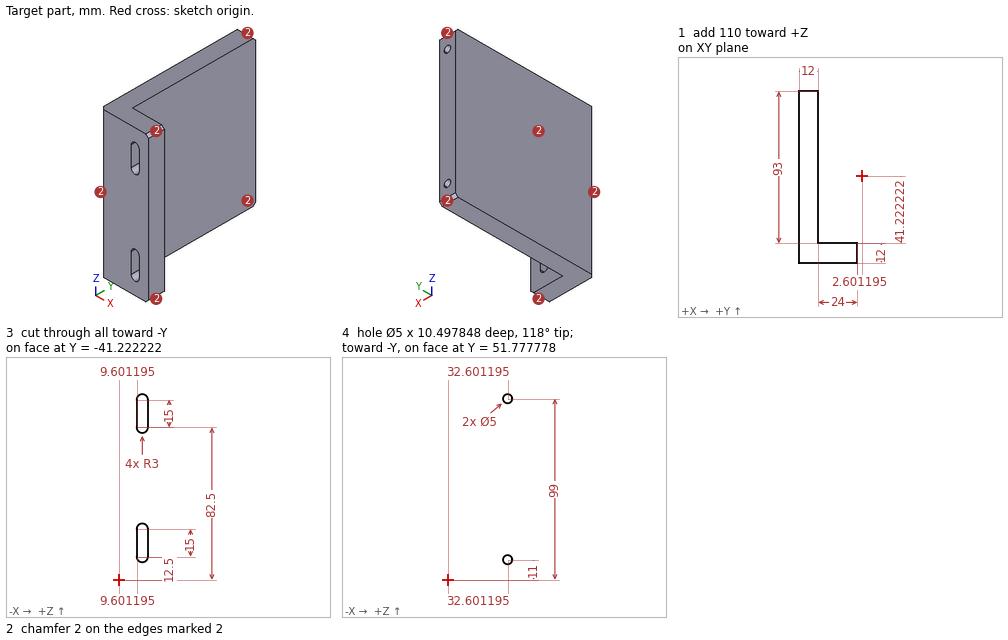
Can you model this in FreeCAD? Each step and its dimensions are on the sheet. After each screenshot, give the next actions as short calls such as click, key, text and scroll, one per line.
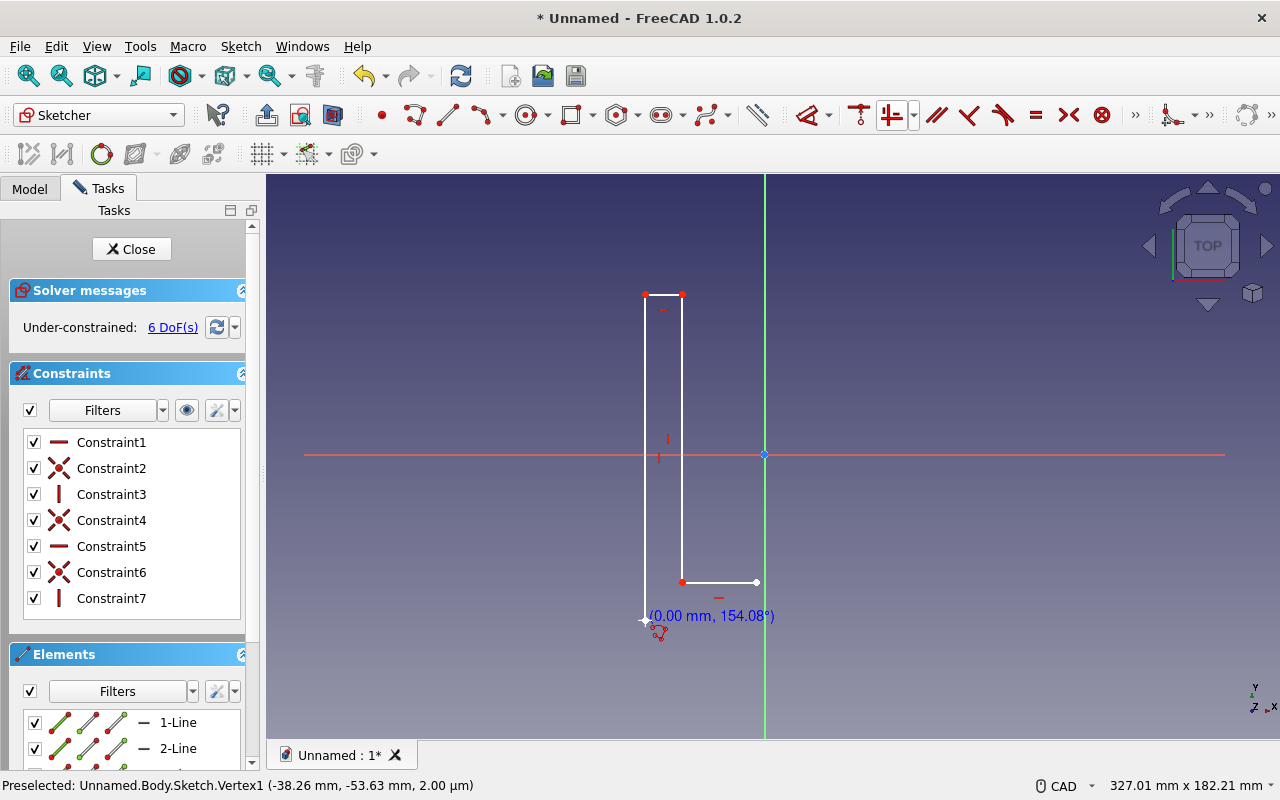
scroll(757, 620, up, 4)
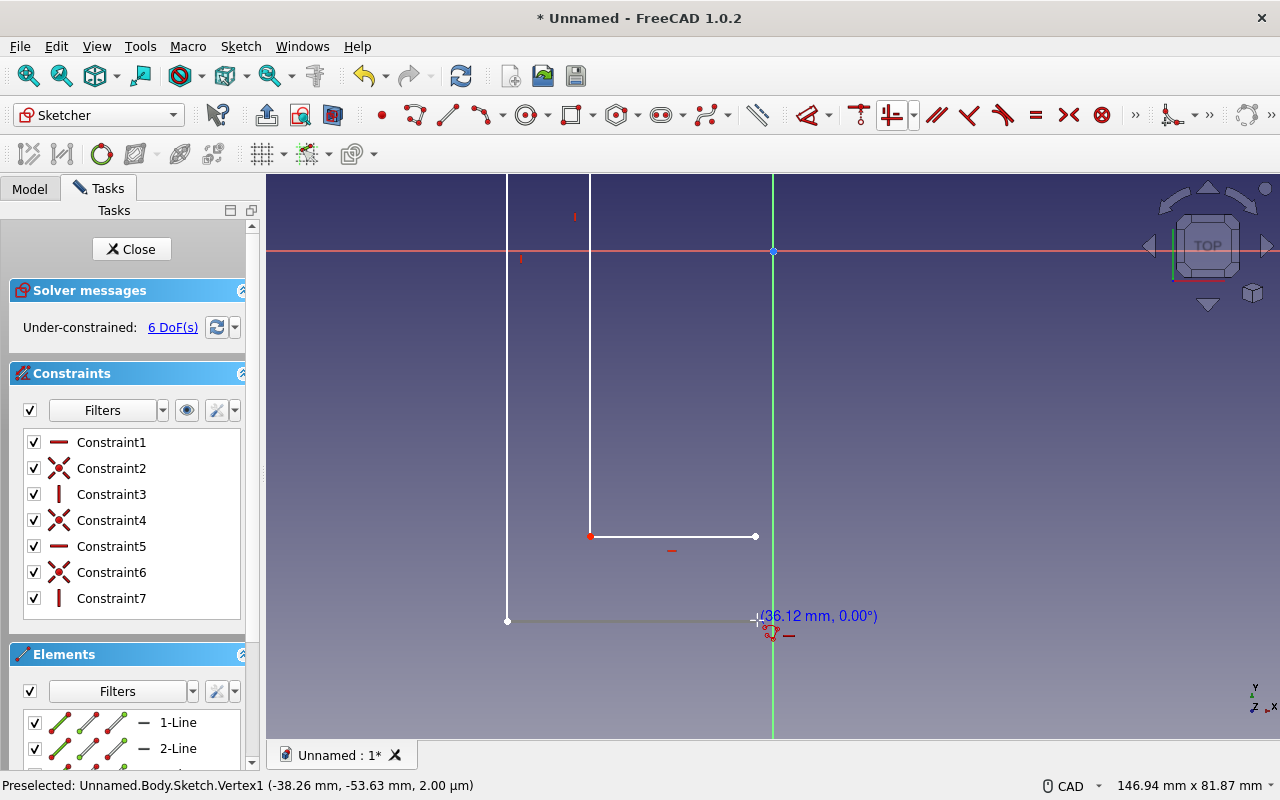
click(755, 619)
click(755, 537)
key(Escape)
key(Escape)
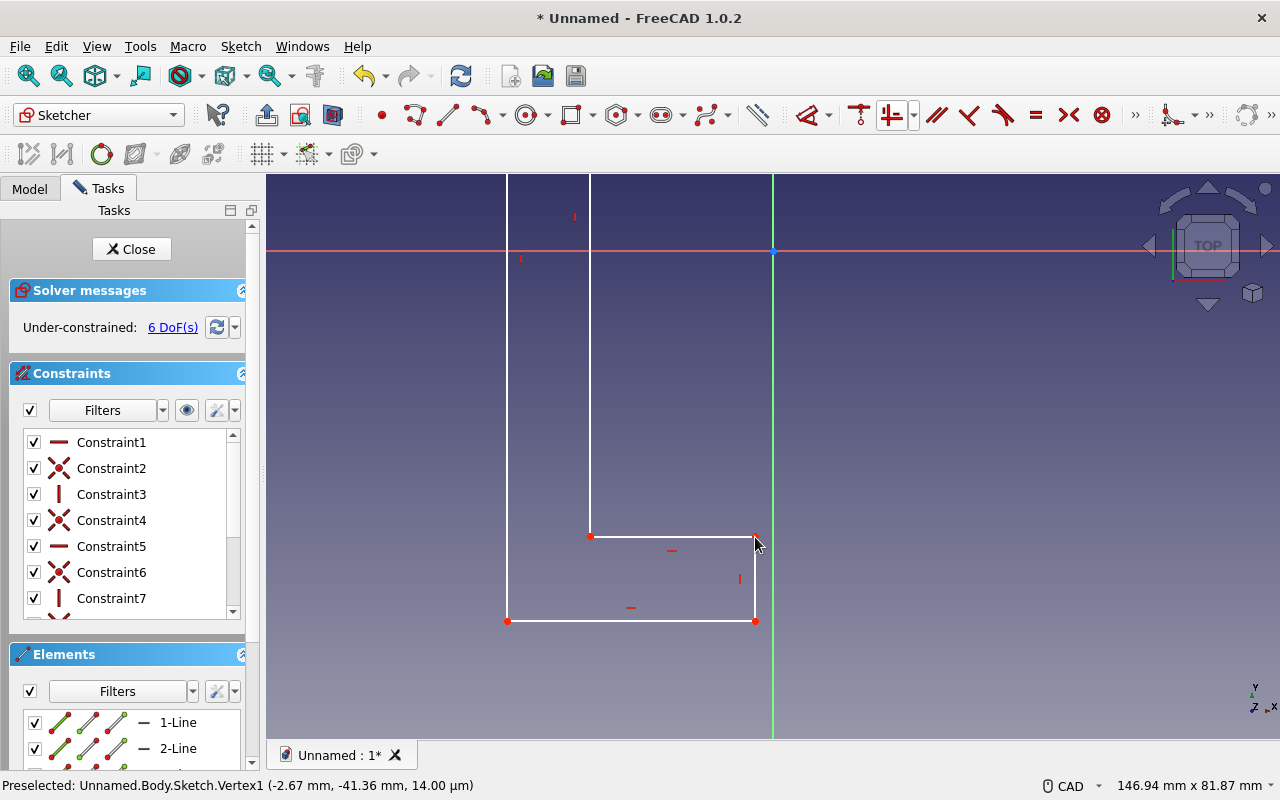
click(806, 116)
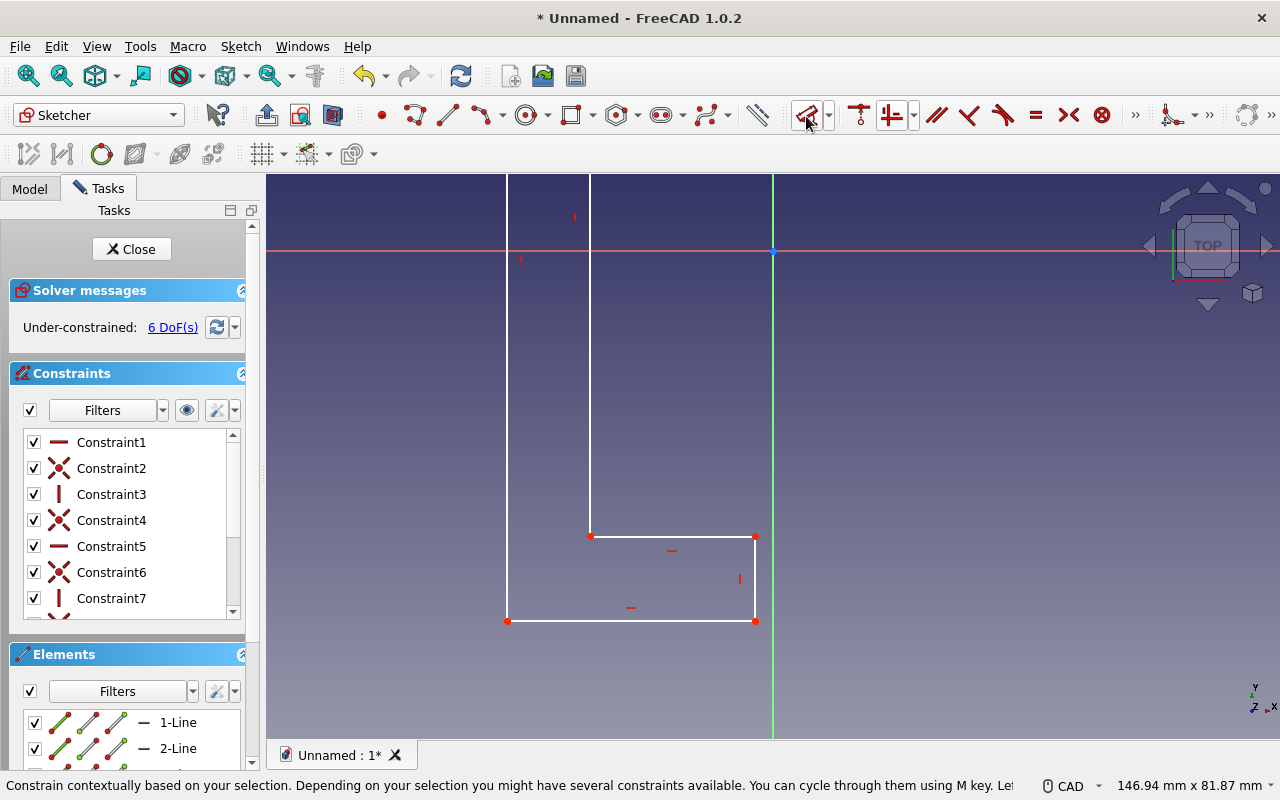
click(705, 537)
click(672, 571)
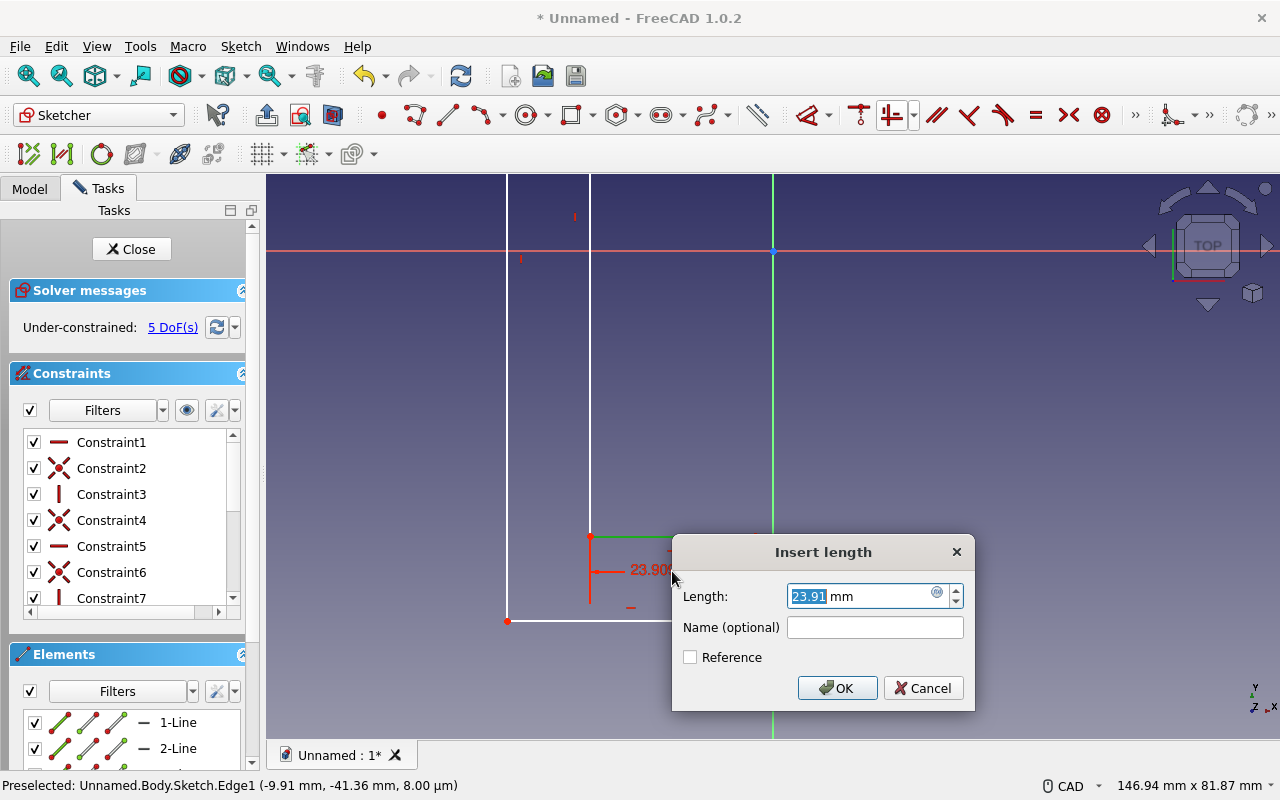
text(24)
key(Return)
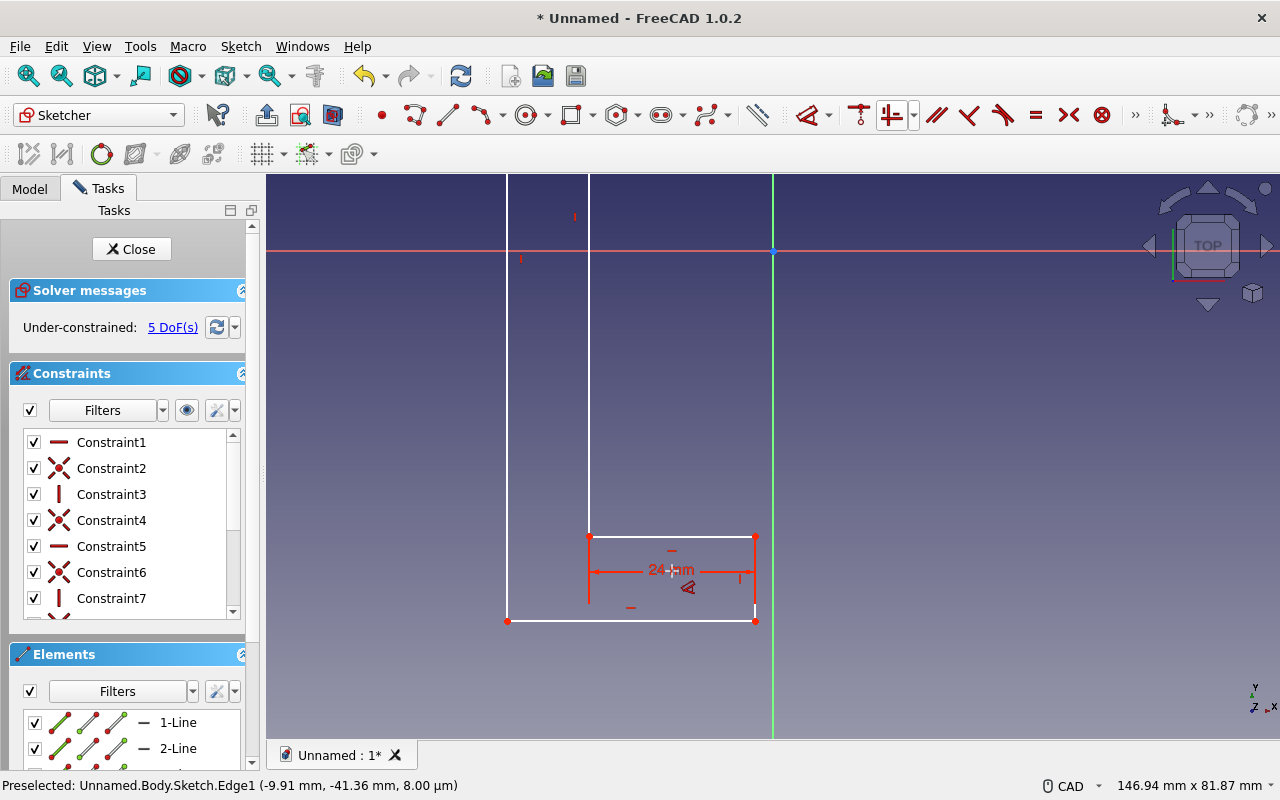
click(589, 344)
click(555, 369)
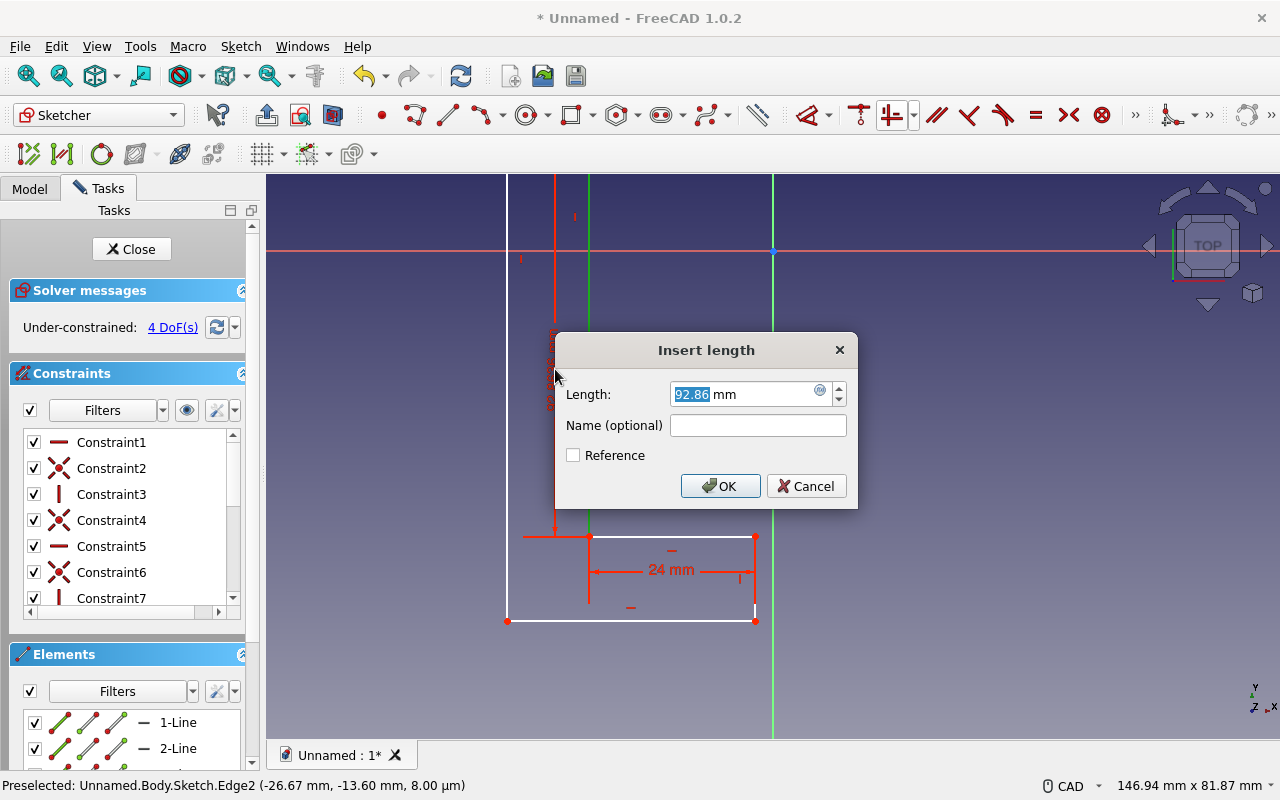
text(93)
key(Return)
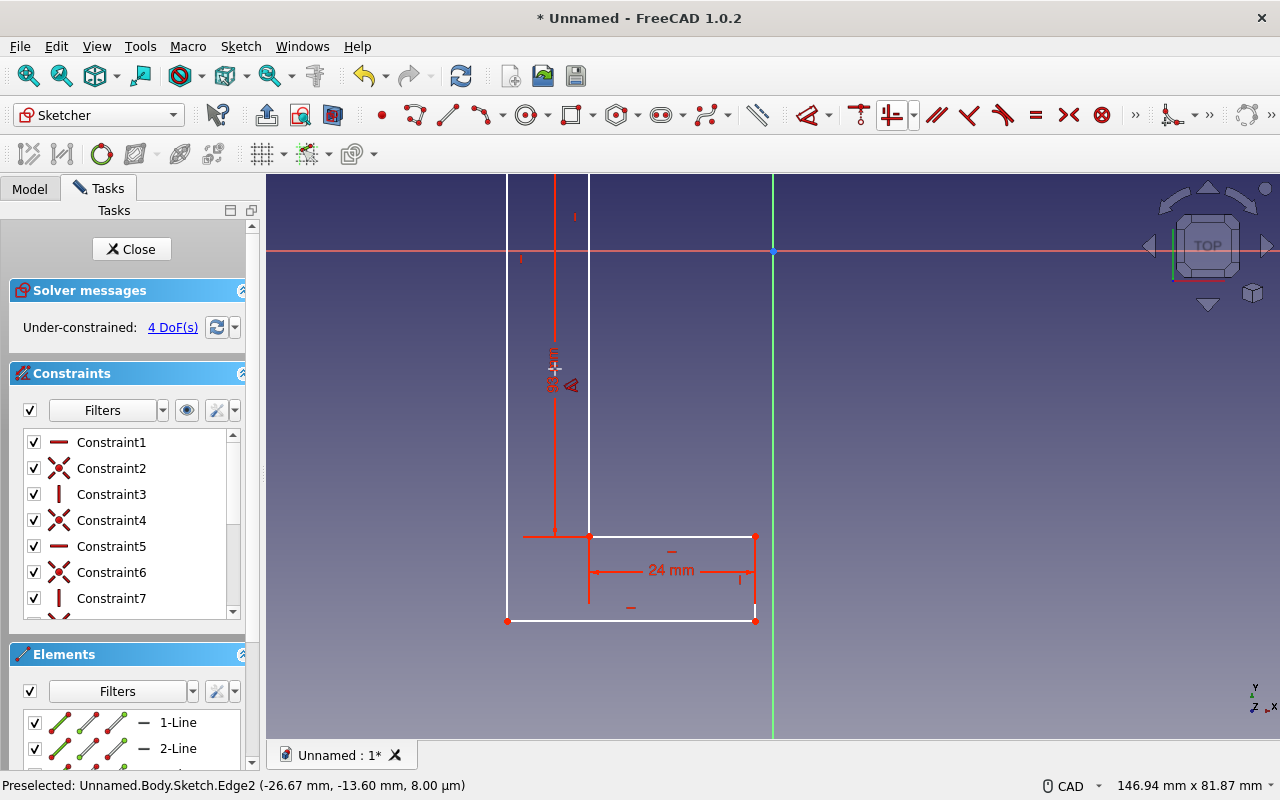
scroll(757, 620, down, 4)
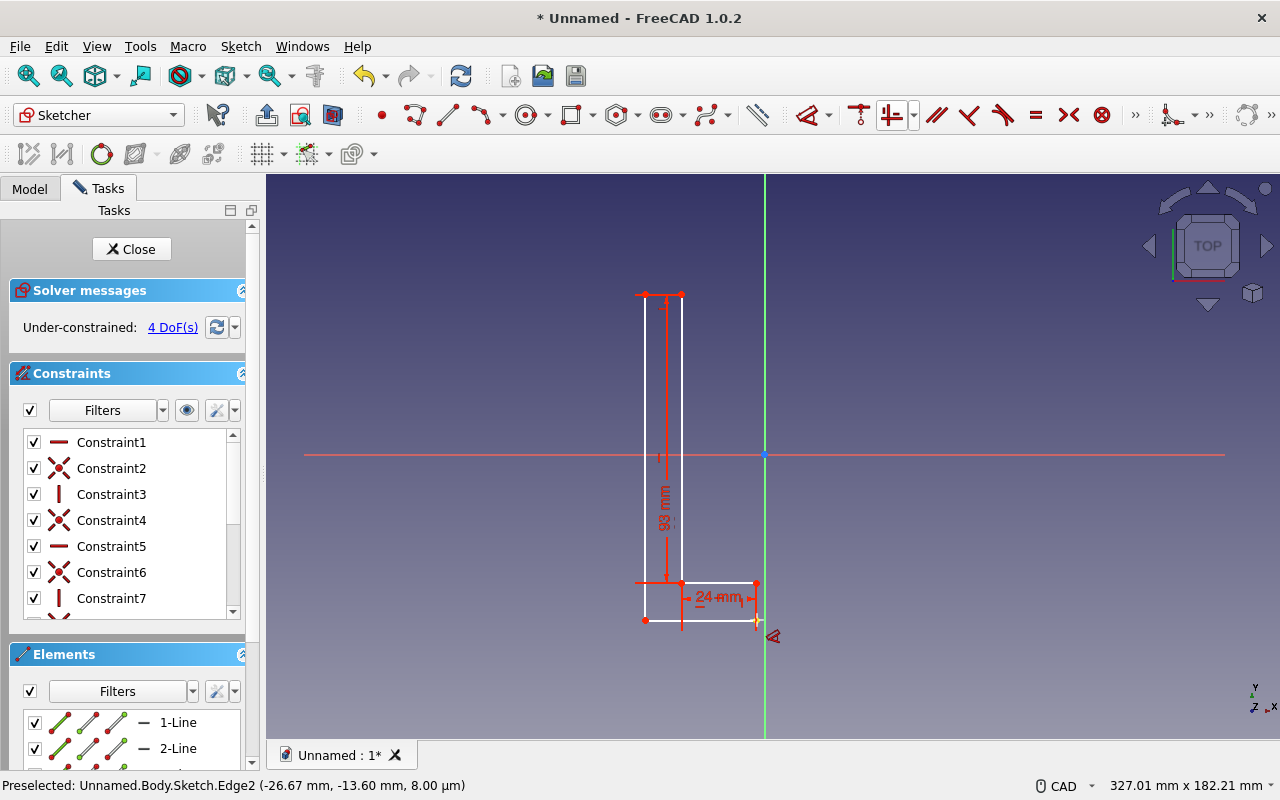
scroll(671, 295, up, 2)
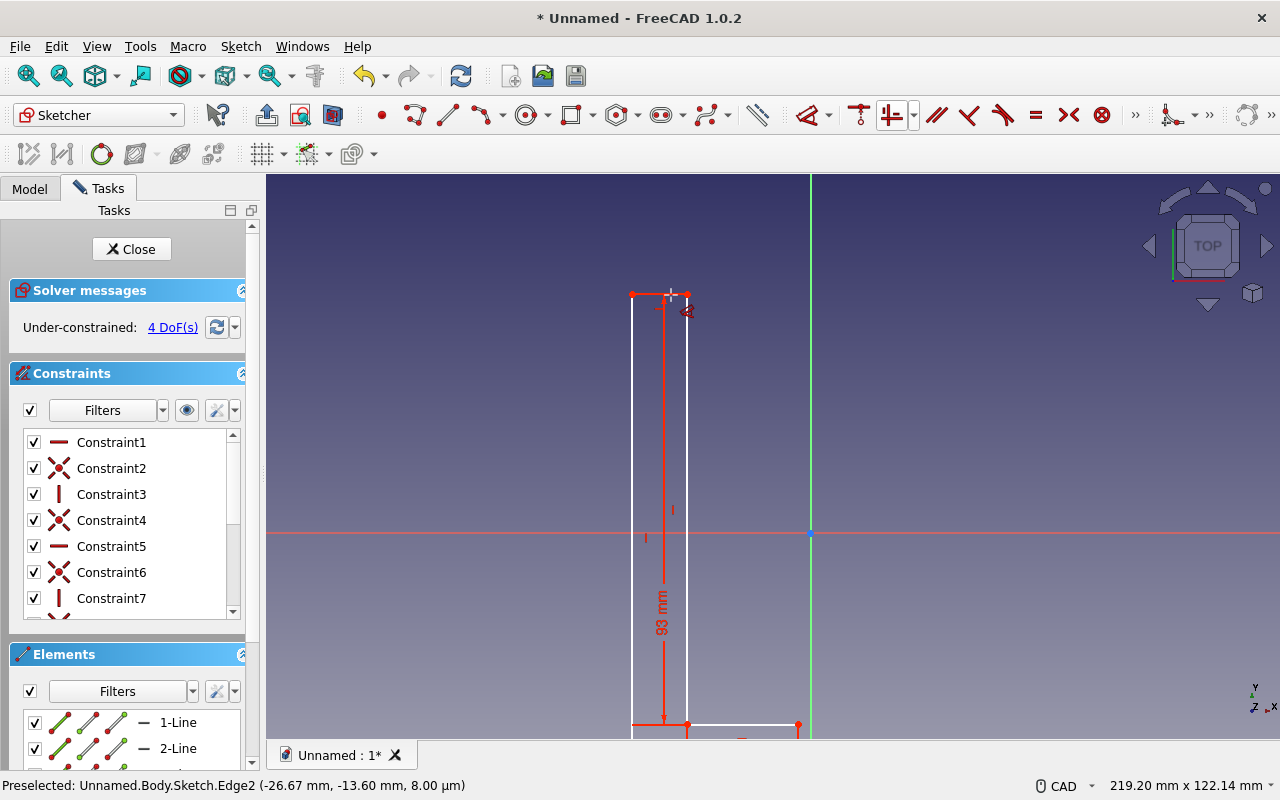
click(671, 294)
click(660, 260)